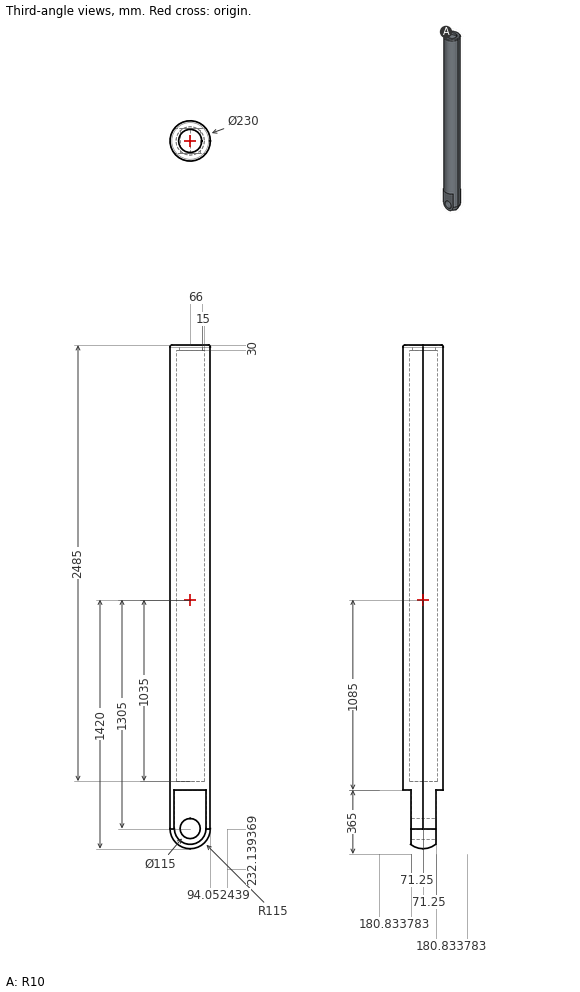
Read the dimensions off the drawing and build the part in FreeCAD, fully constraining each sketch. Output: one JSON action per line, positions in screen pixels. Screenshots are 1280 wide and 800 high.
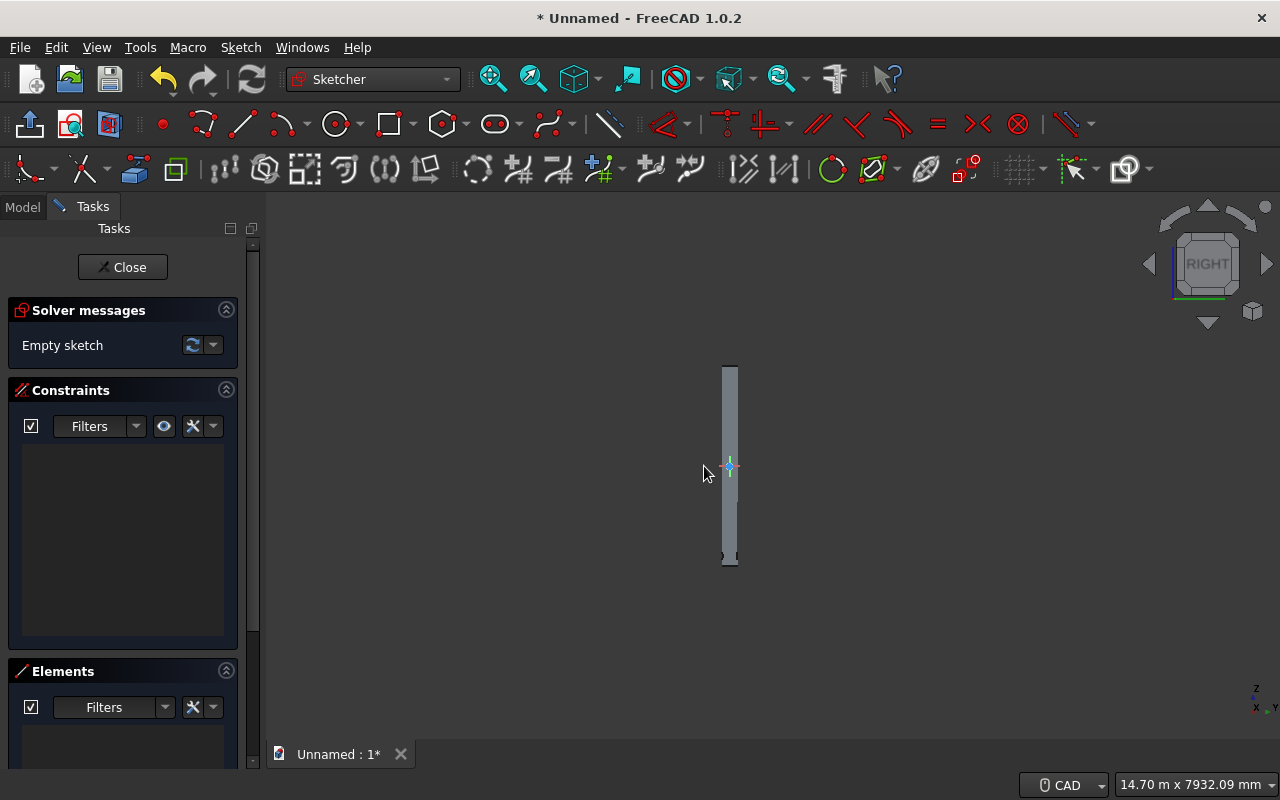
{"action": "scroll", "coordinate": [732, 561], "scroll_direction": "up", "scroll_amount": 13}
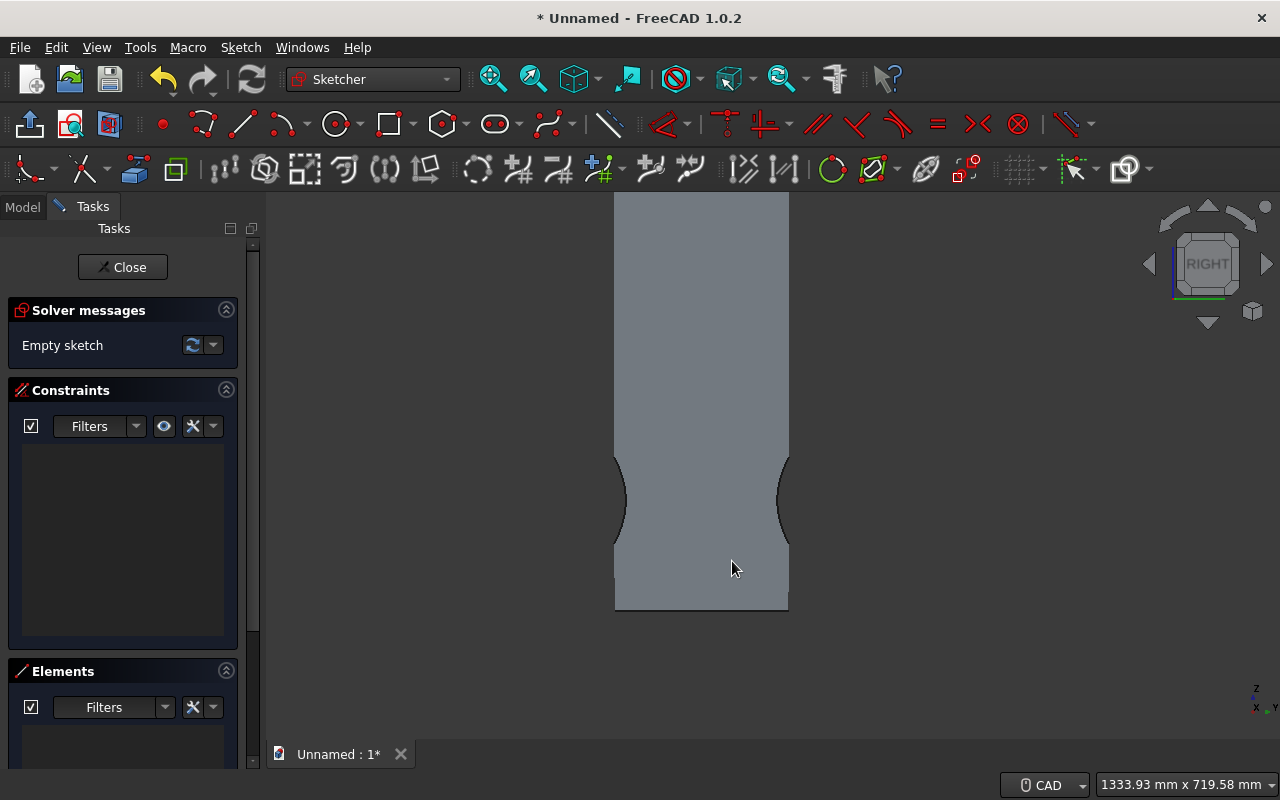
{"action": "left_click", "coordinate": [390, 124]}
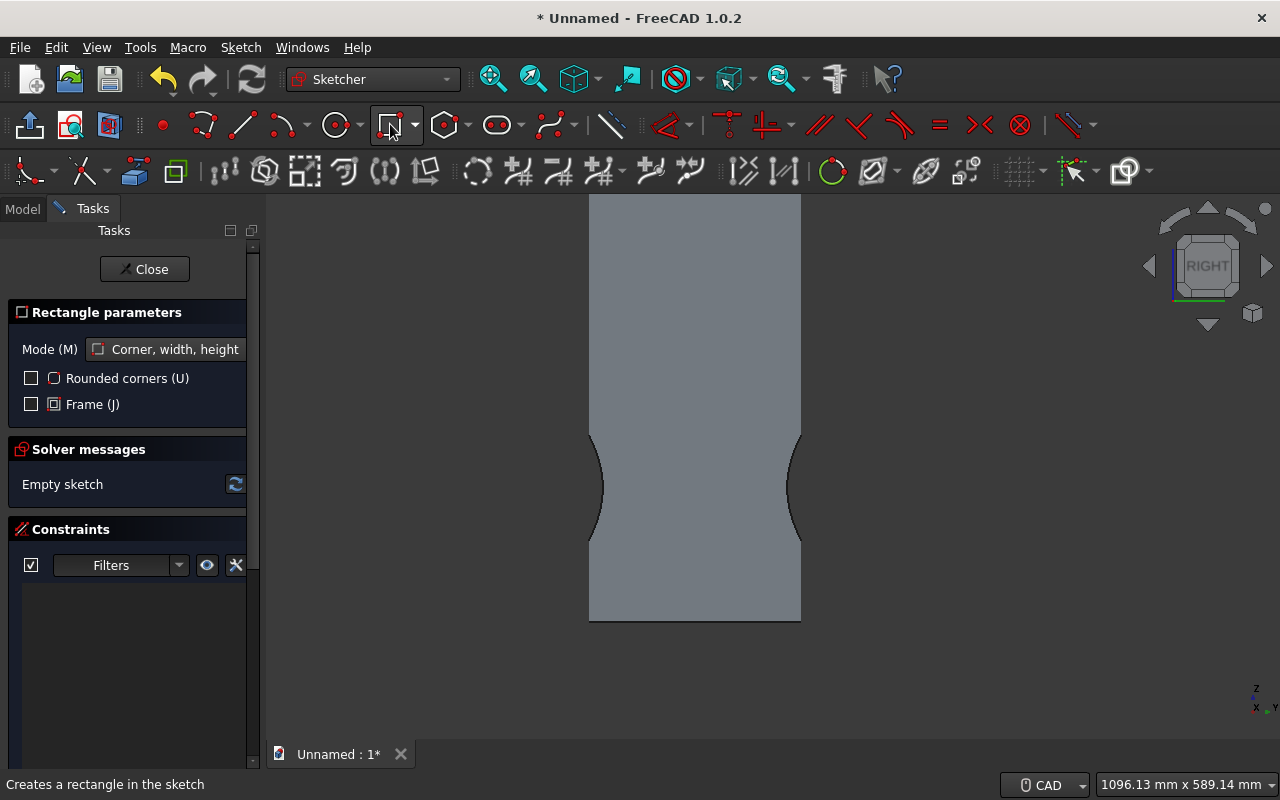
{"action": "left_click", "coordinate": [462, 284]}
{"action": "mouse_move", "coordinate": [629, 622]}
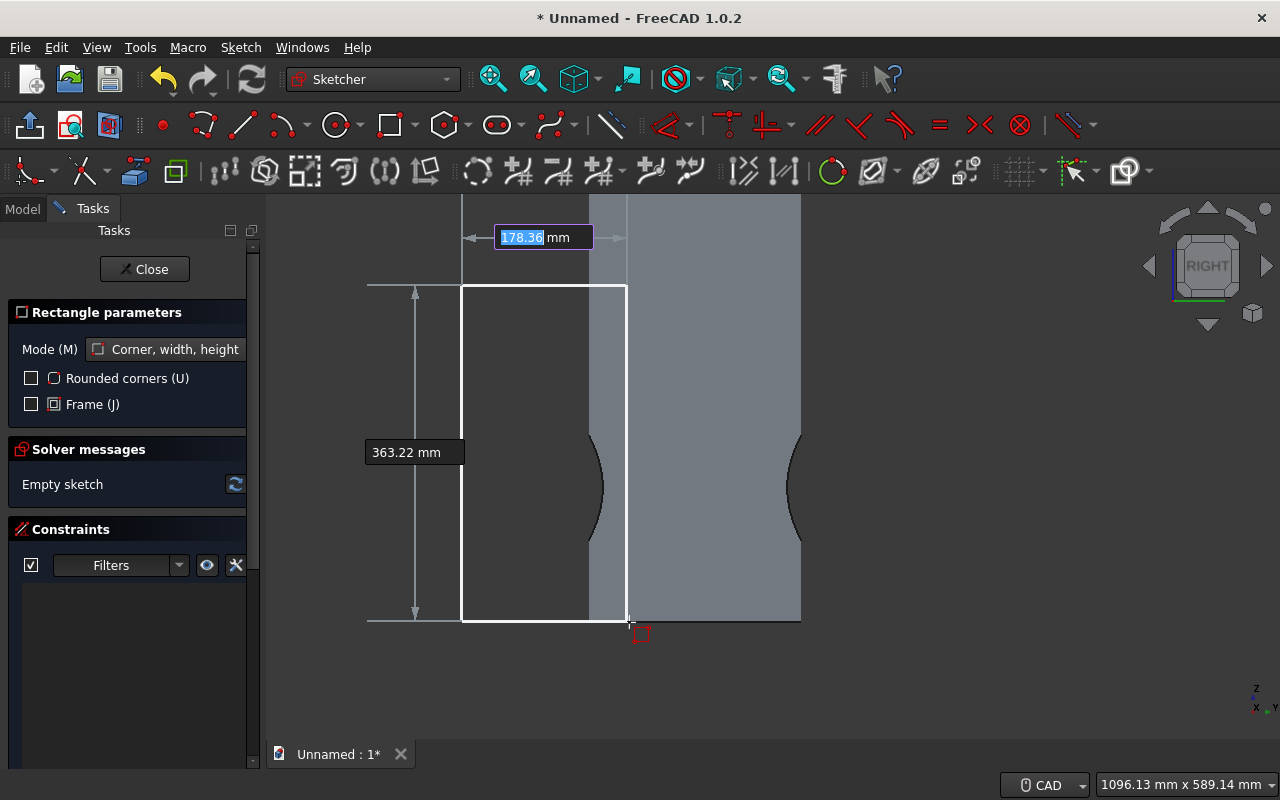
{"action": "type", "text": "180.833783"}
{"action": "key", "text": "Tab"}
{"action": "type", "text": "365"}
{"action": "key", "text": "Return"}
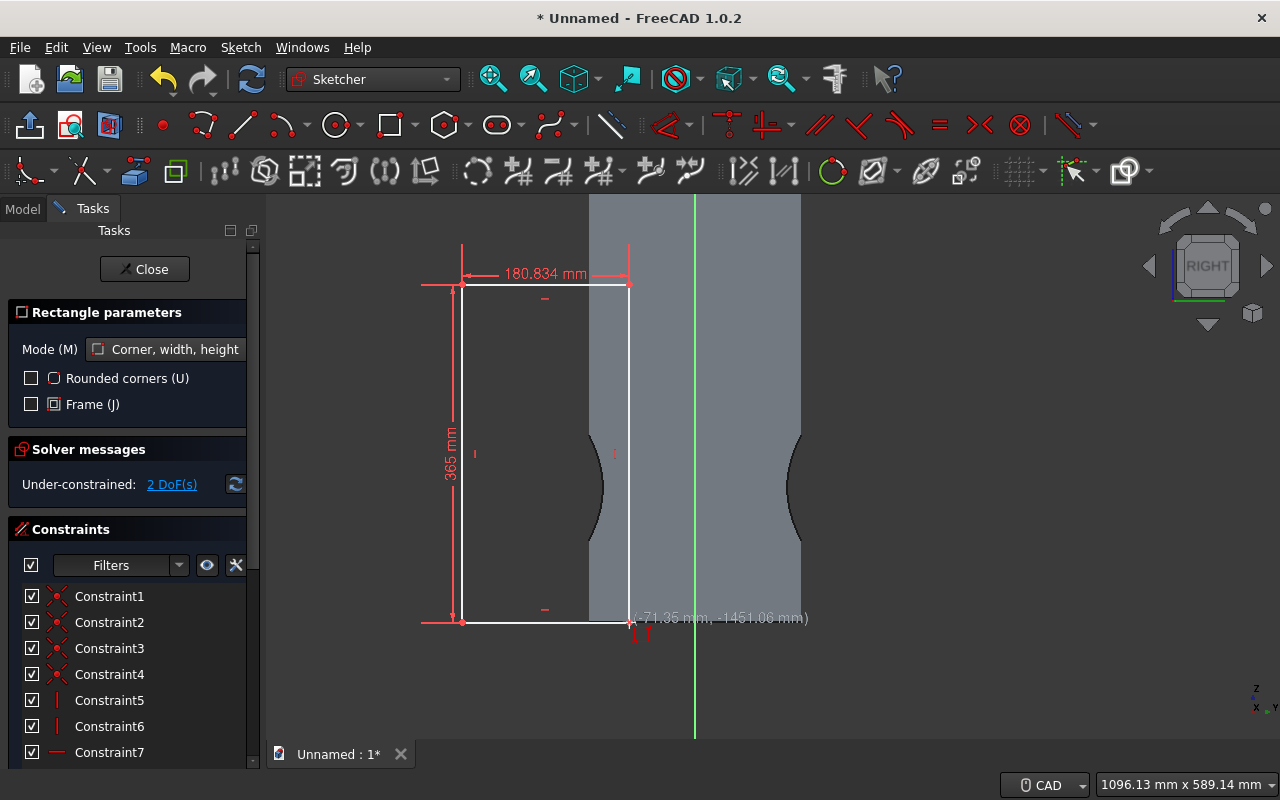
{"action": "left_click", "coordinate": [761, 284]}
{"action": "mouse_move", "coordinate": [928, 622]}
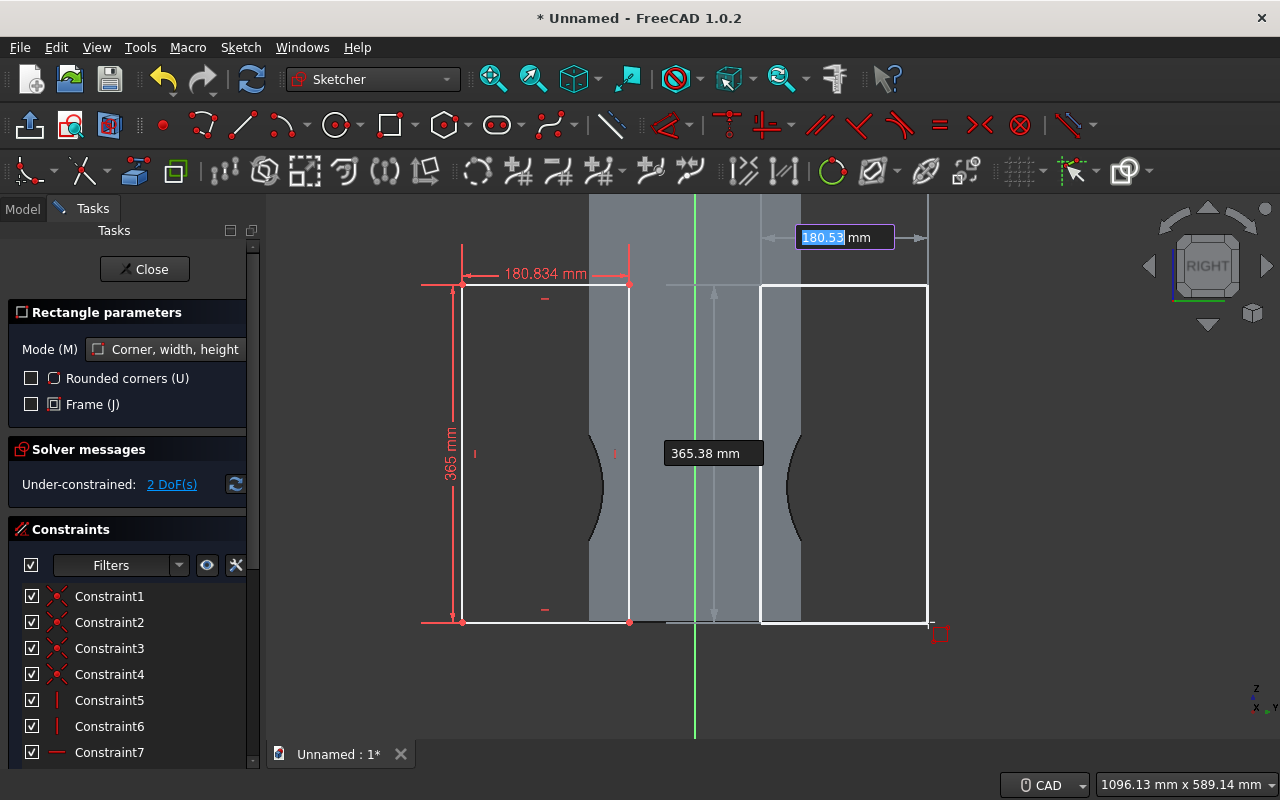
{"action": "type", "text": "180.833783"}
{"action": "key", "text": "Tab"}
{"action": "type", "text": "365"}
{"action": "key", "text": "Return"}
{"action": "key", "text": "Escape"}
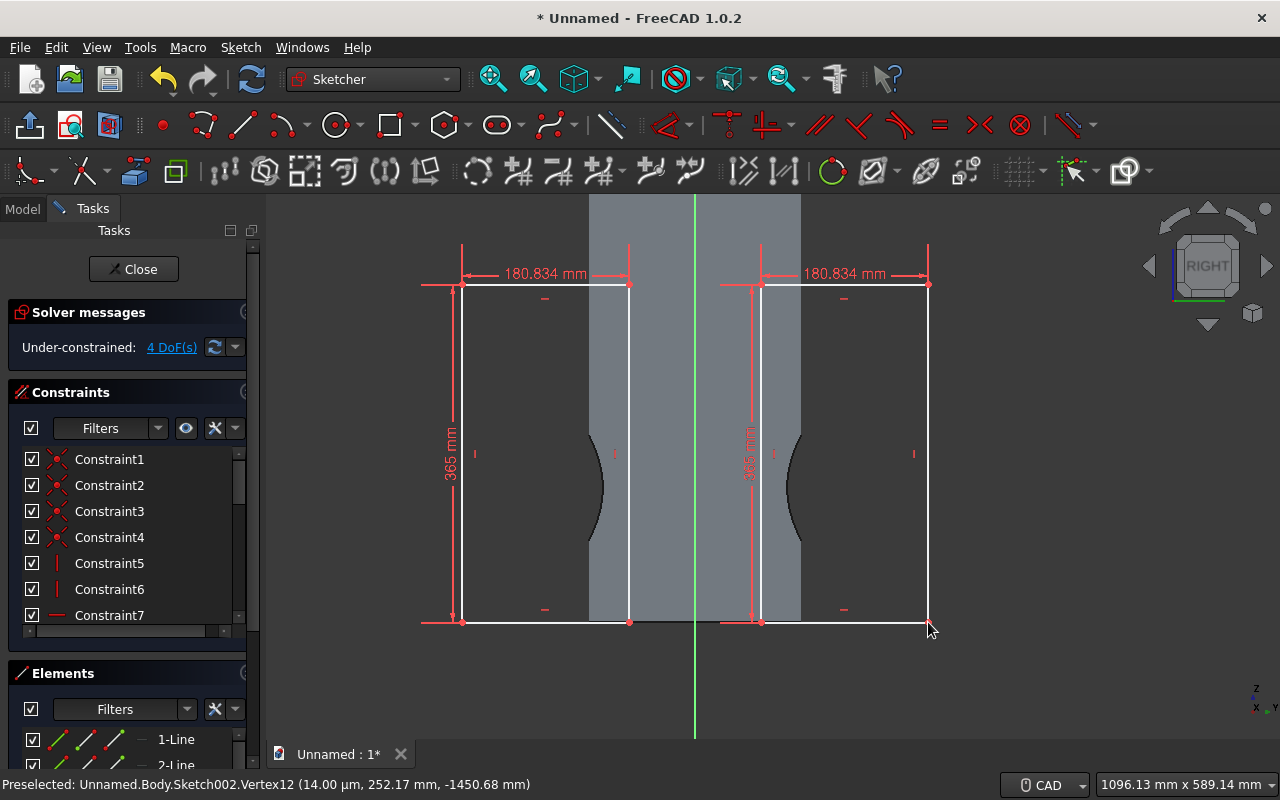
{"action": "left_click", "coordinate": [666, 126]}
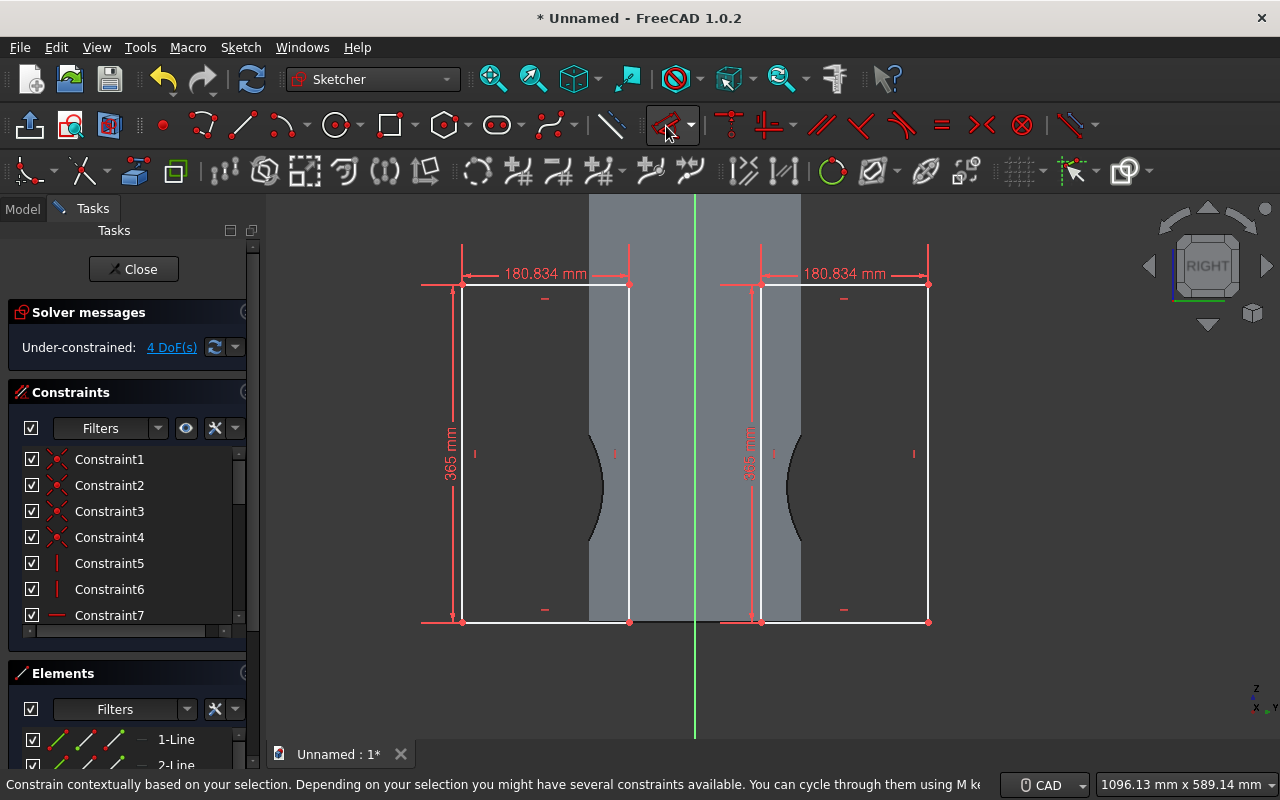
{"action": "left_click", "coordinate": [462, 285]}
{"action": "left_click", "coordinate": [428, 254]}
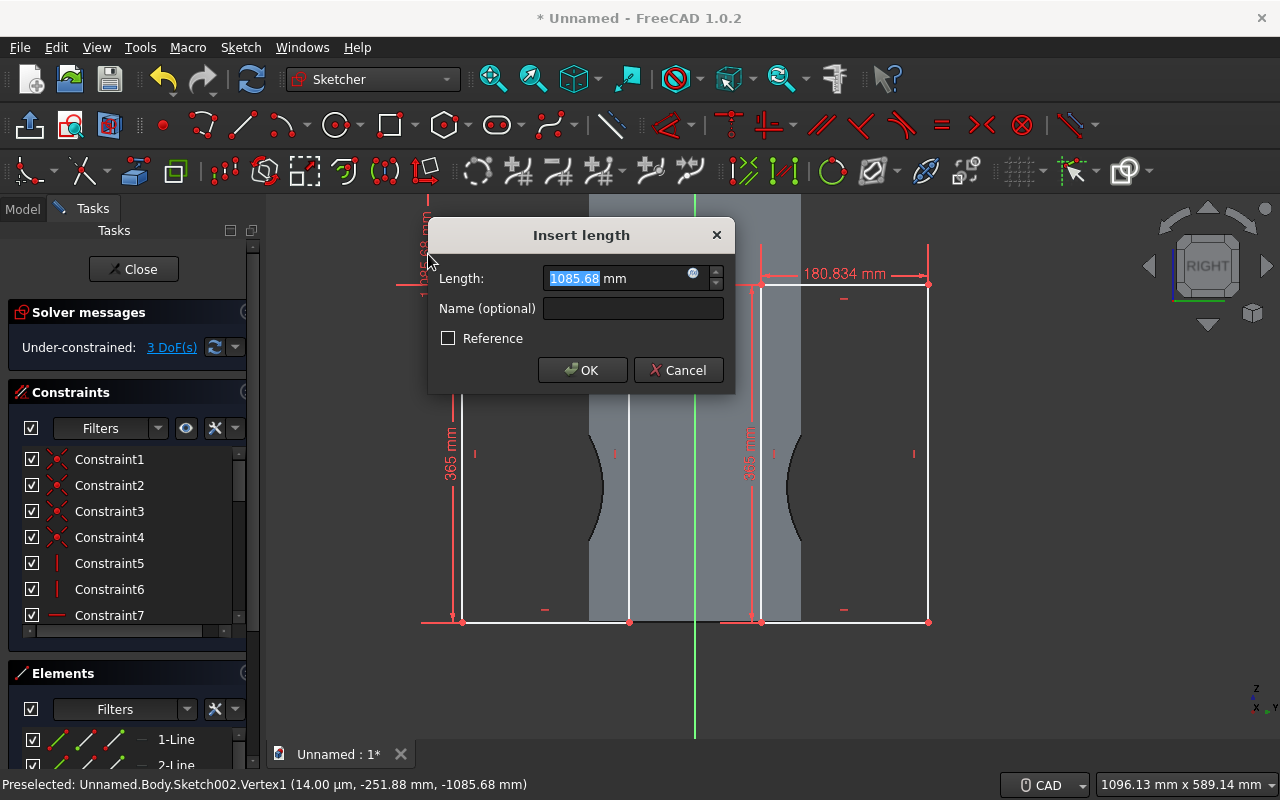
{"action": "type", "text": "1085"}
{"action": "key", "text": "Return"}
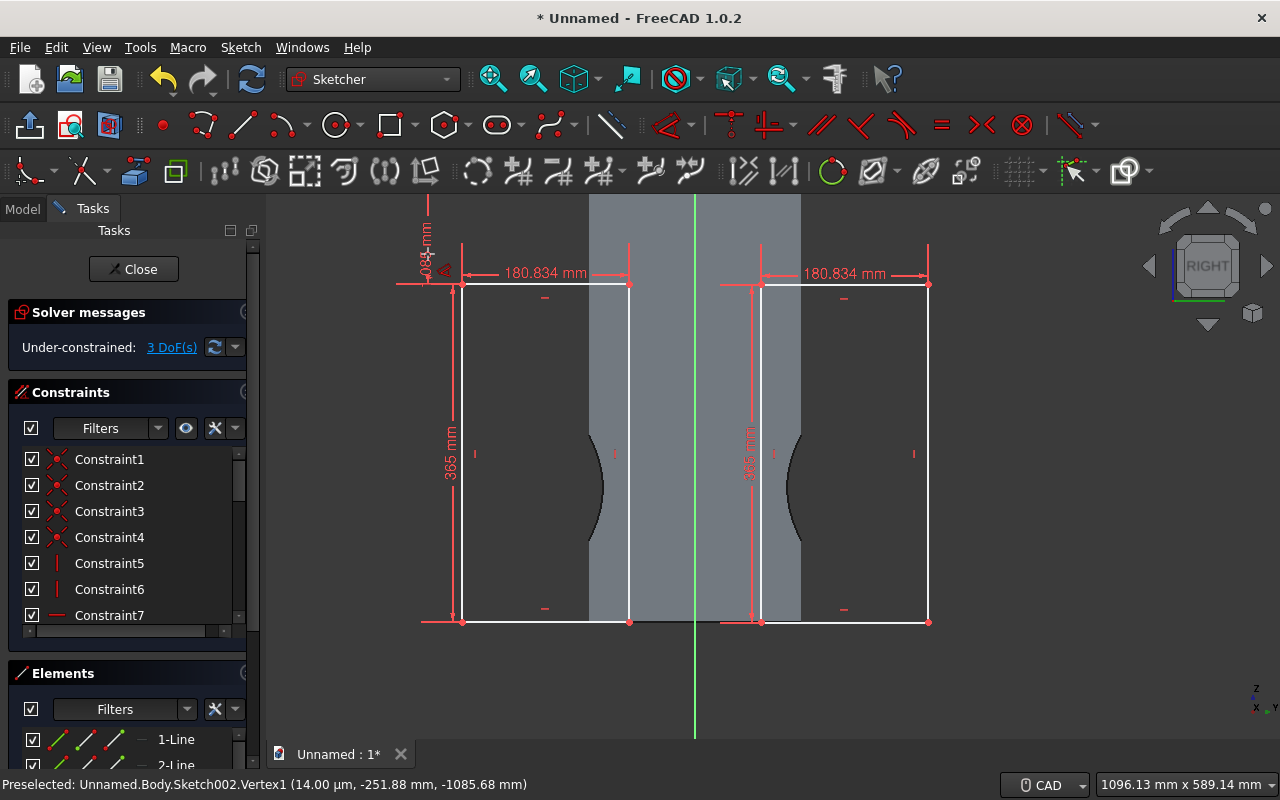
{"action": "left_click", "coordinate": [761, 285]}
{"action": "left_click", "coordinate": [795, 254]}